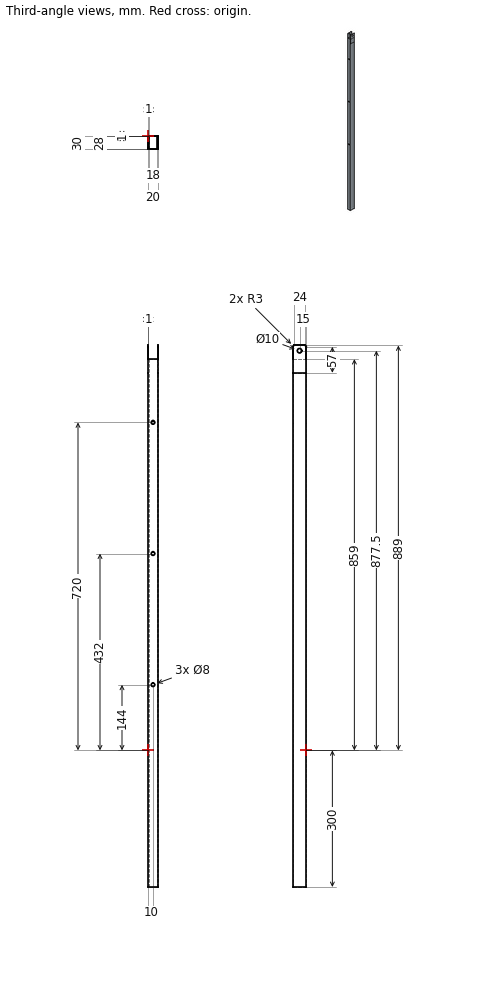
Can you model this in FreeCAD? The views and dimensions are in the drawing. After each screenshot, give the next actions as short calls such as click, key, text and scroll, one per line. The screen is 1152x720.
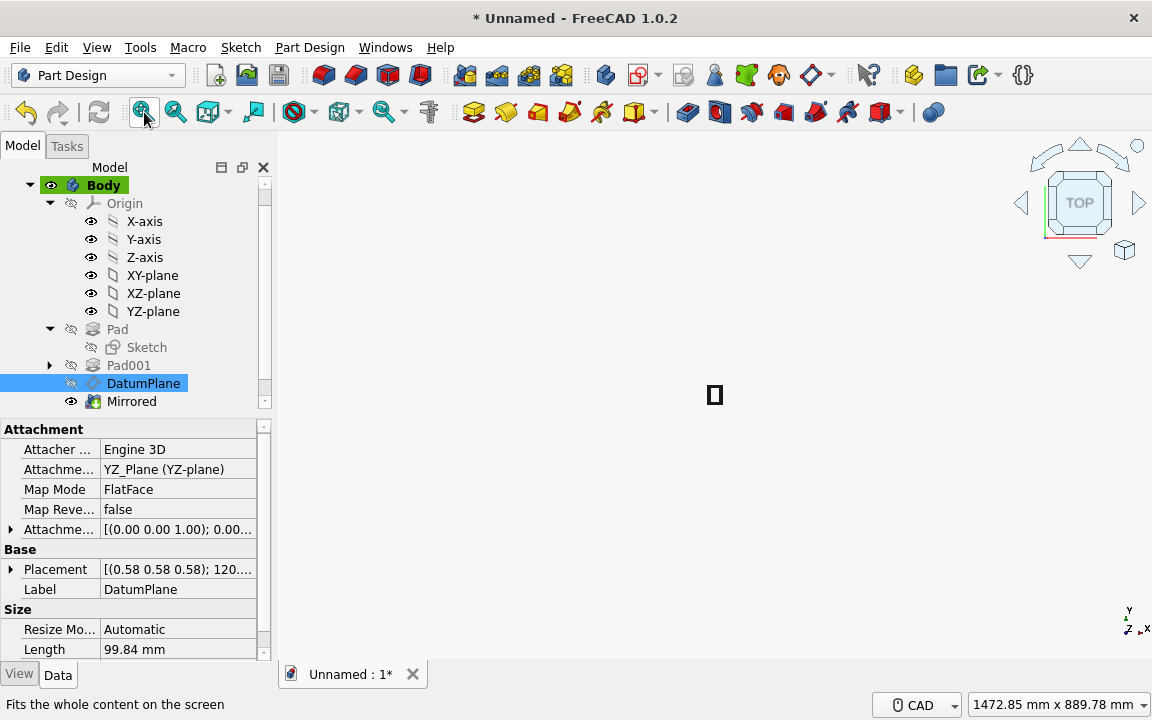
key(v)
key(f)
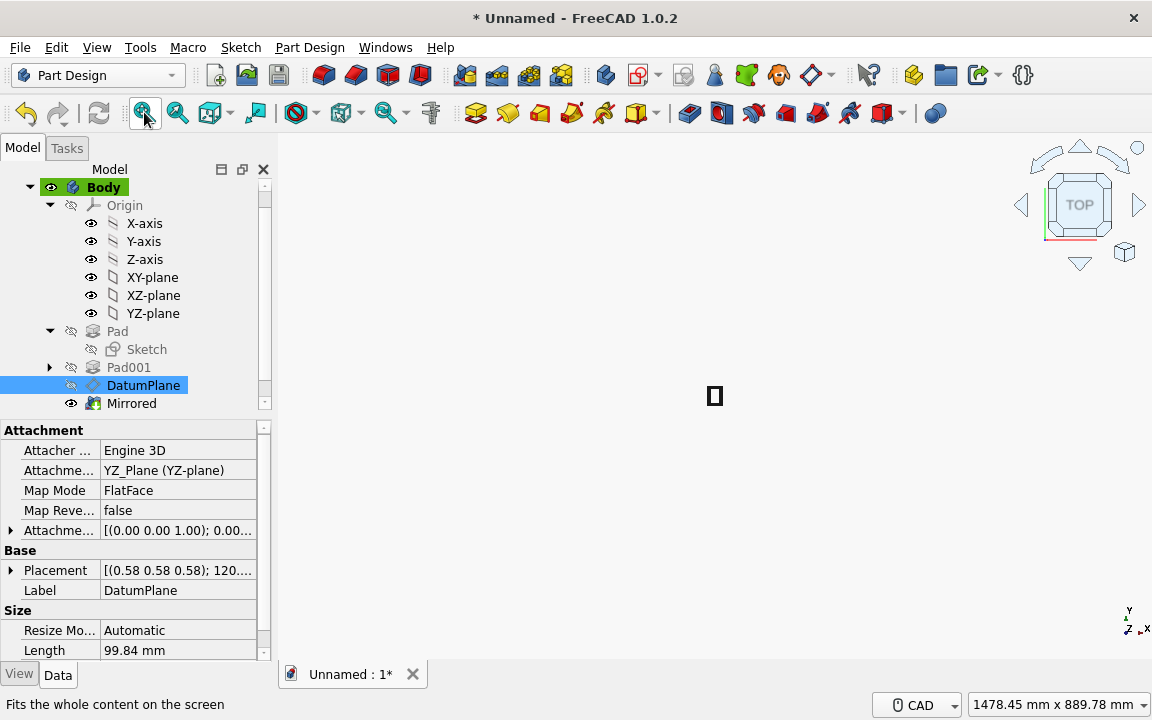
click(136, 313)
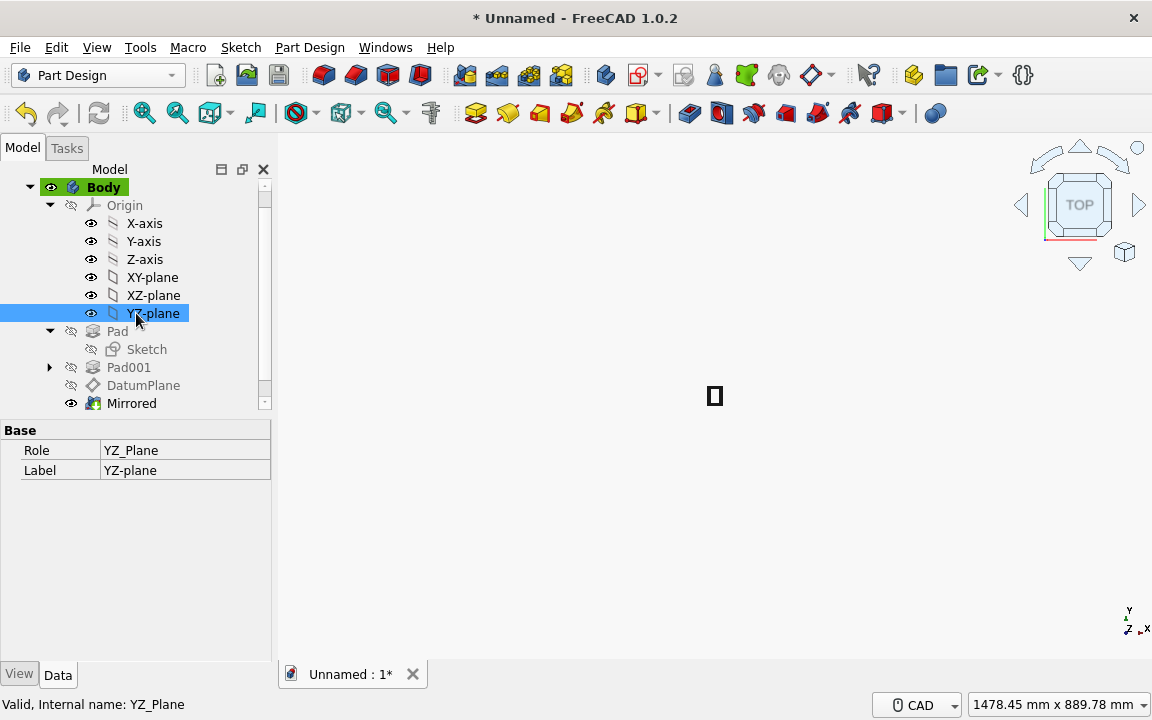
click(812, 76)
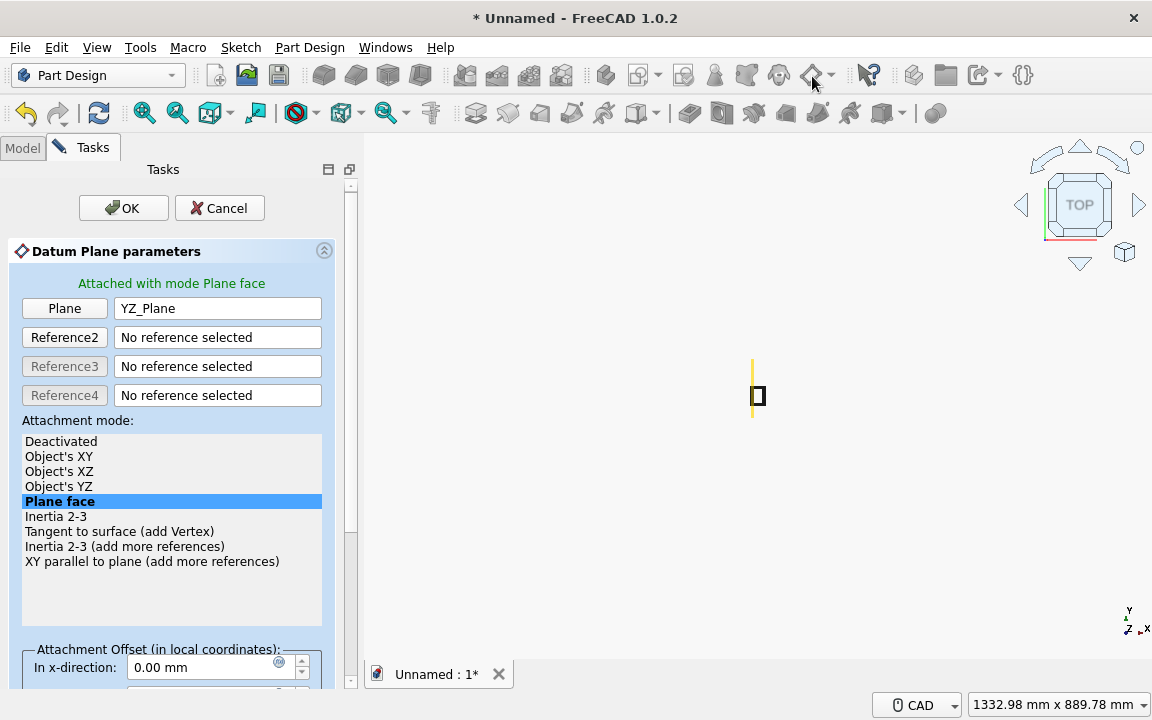
scroll(351, 434, down, 2)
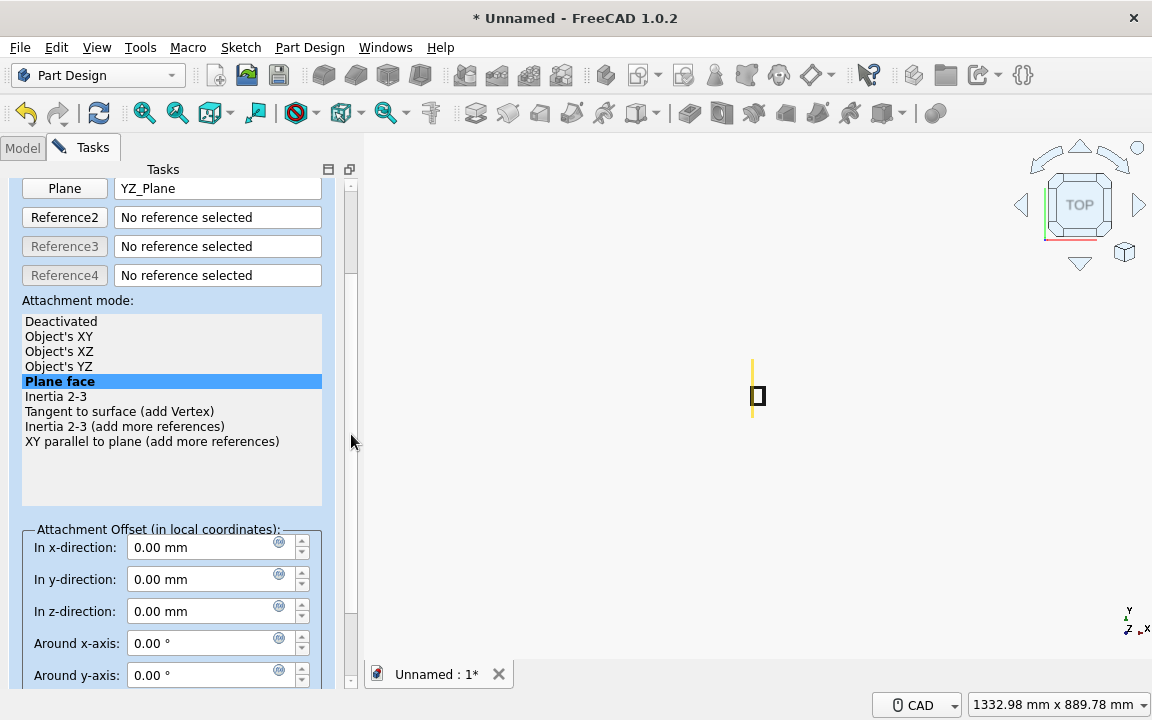
triple_click(210, 611)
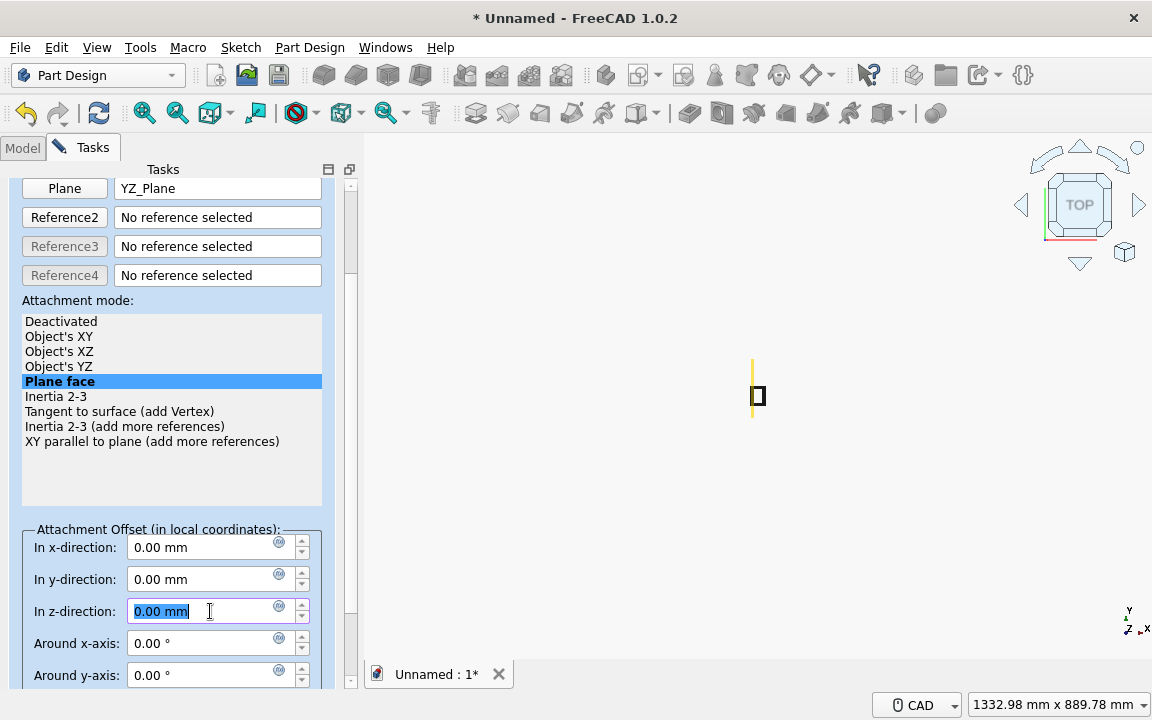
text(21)
key(Tab)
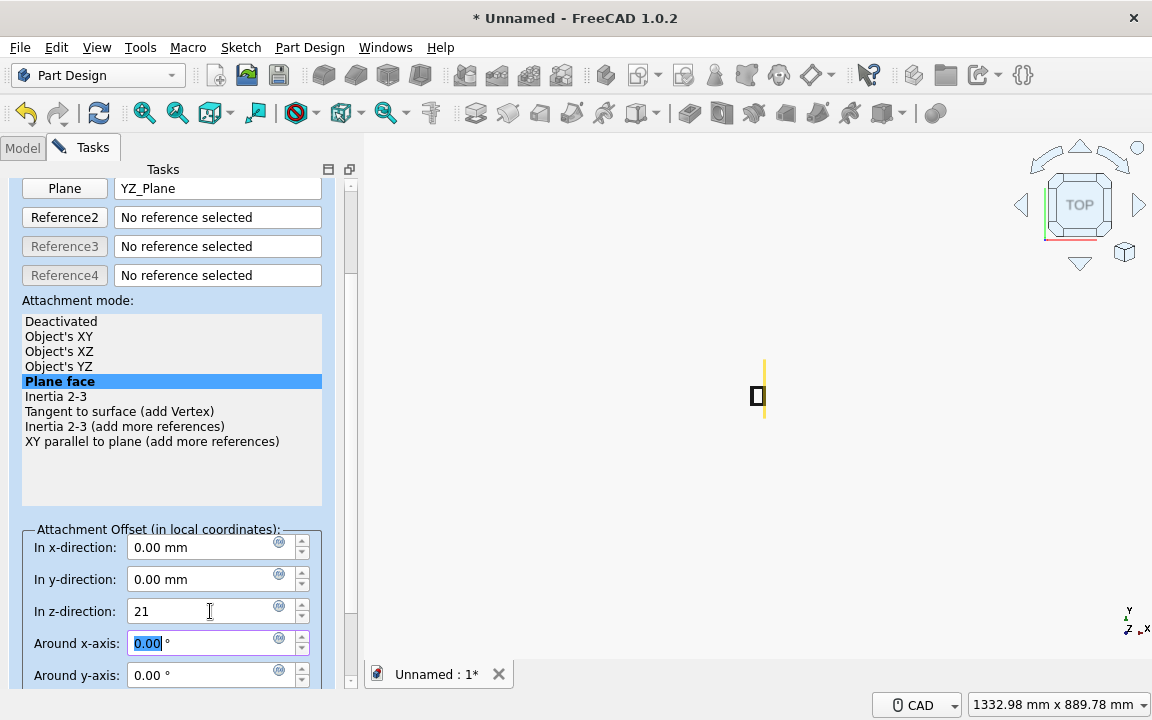
scroll(351, 434, up, 3)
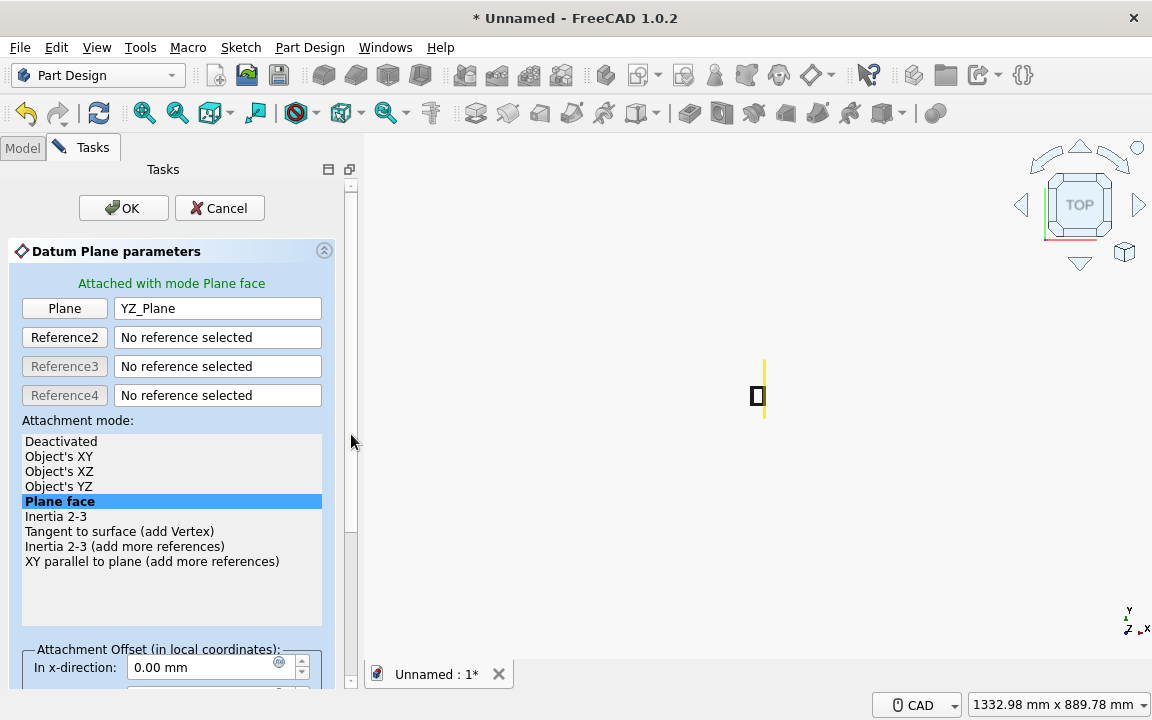
click(124, 208)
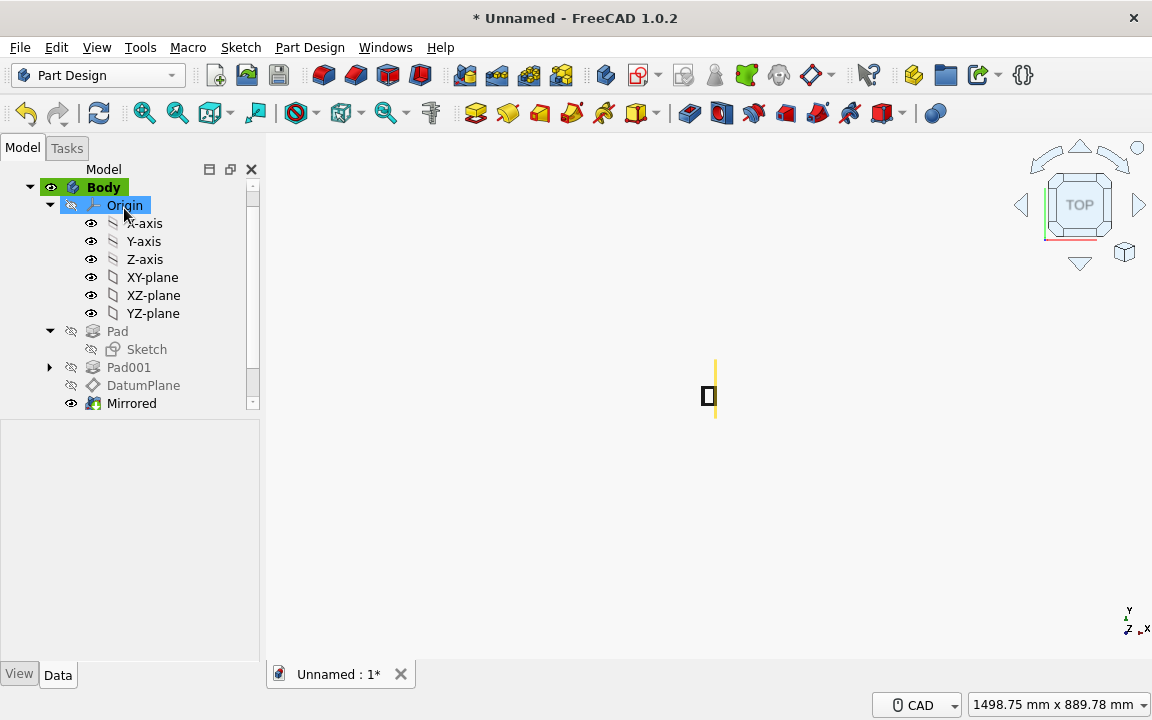
scroll(120, 291, down, 3)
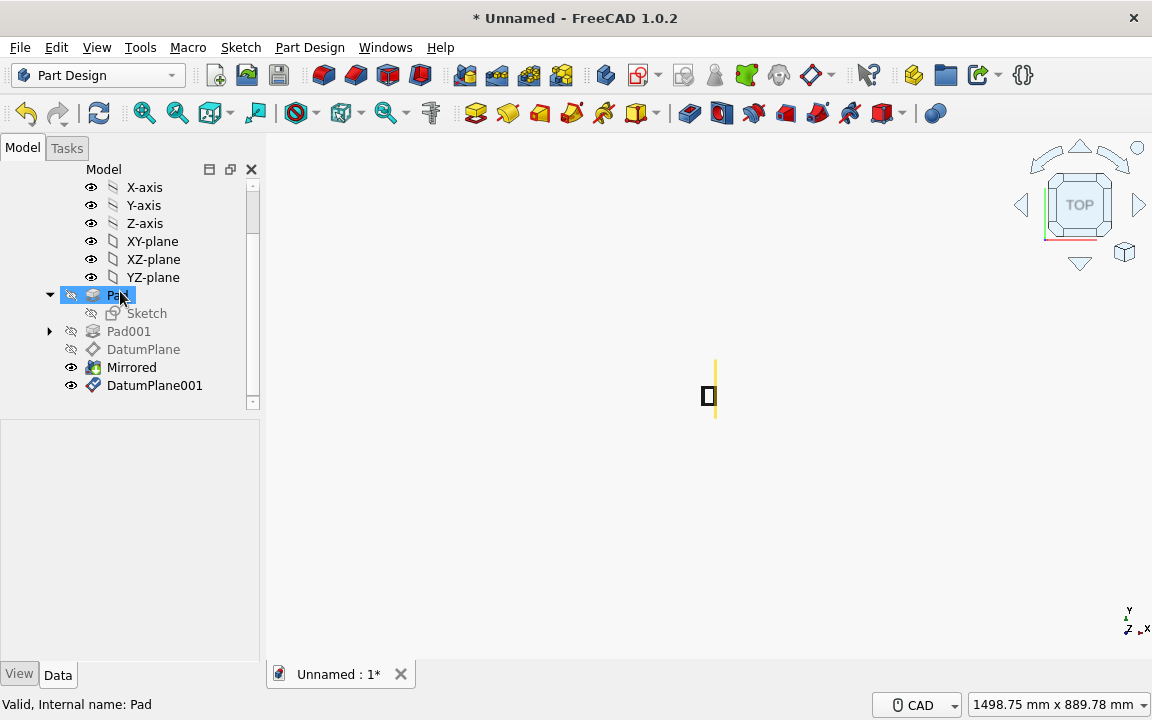
click(116, 385)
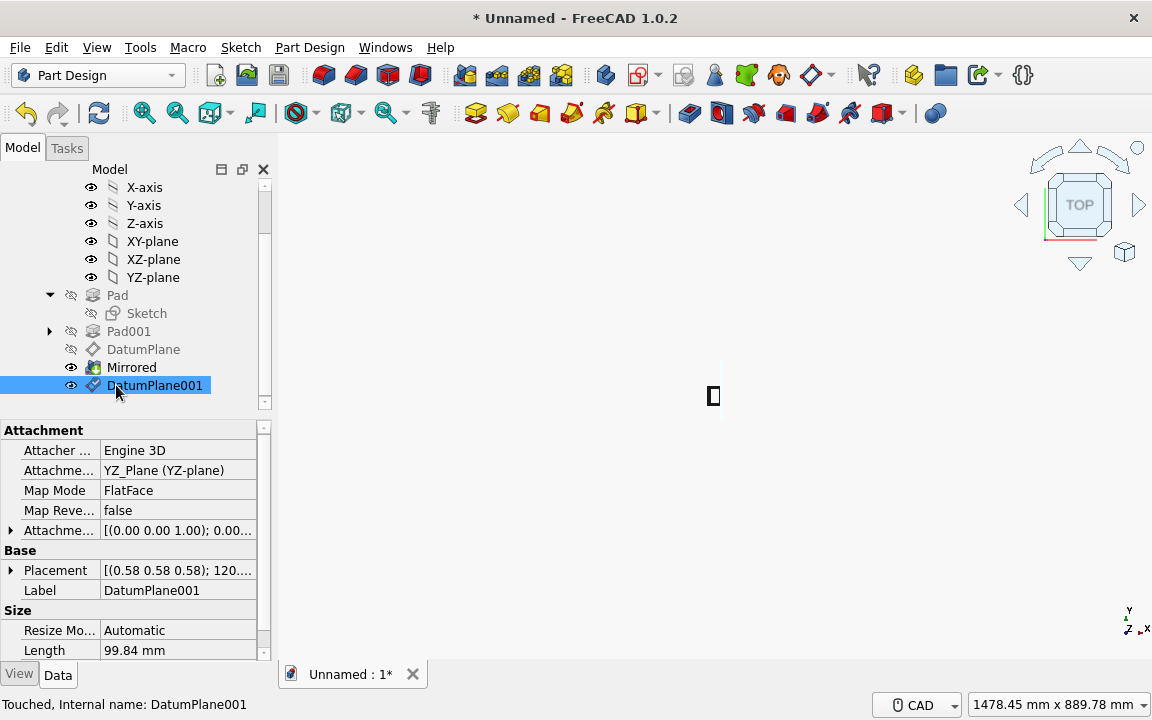
click(638, 76)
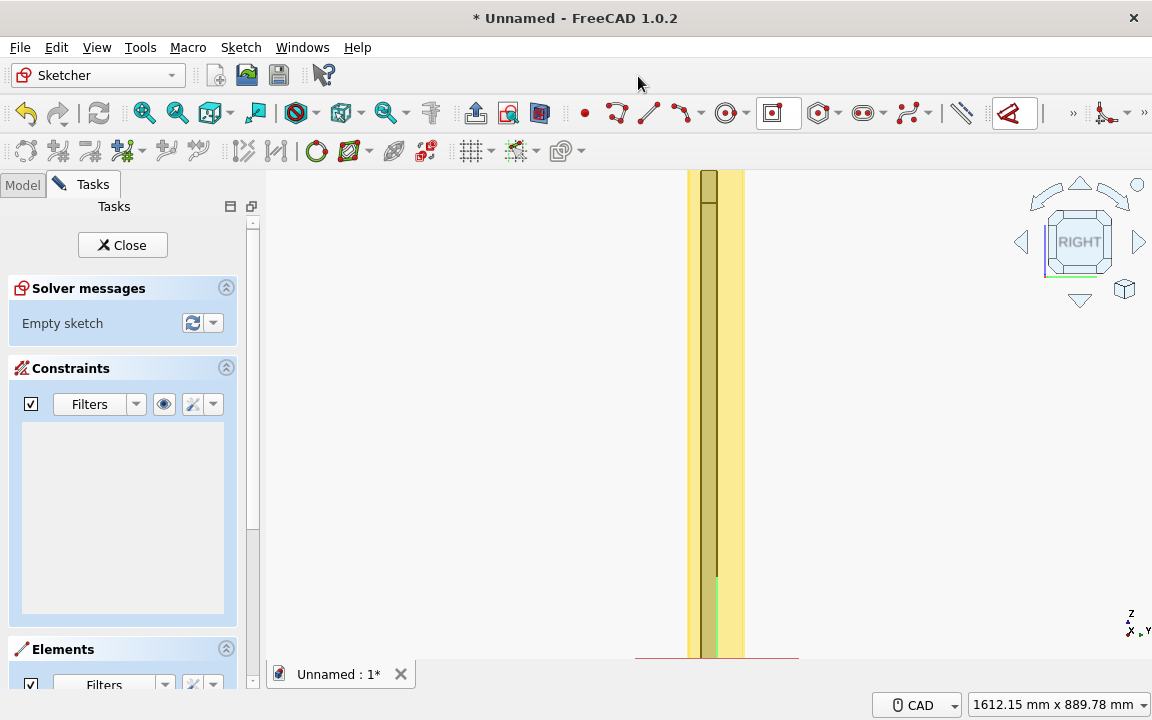
scroll(640, 414, down, 5)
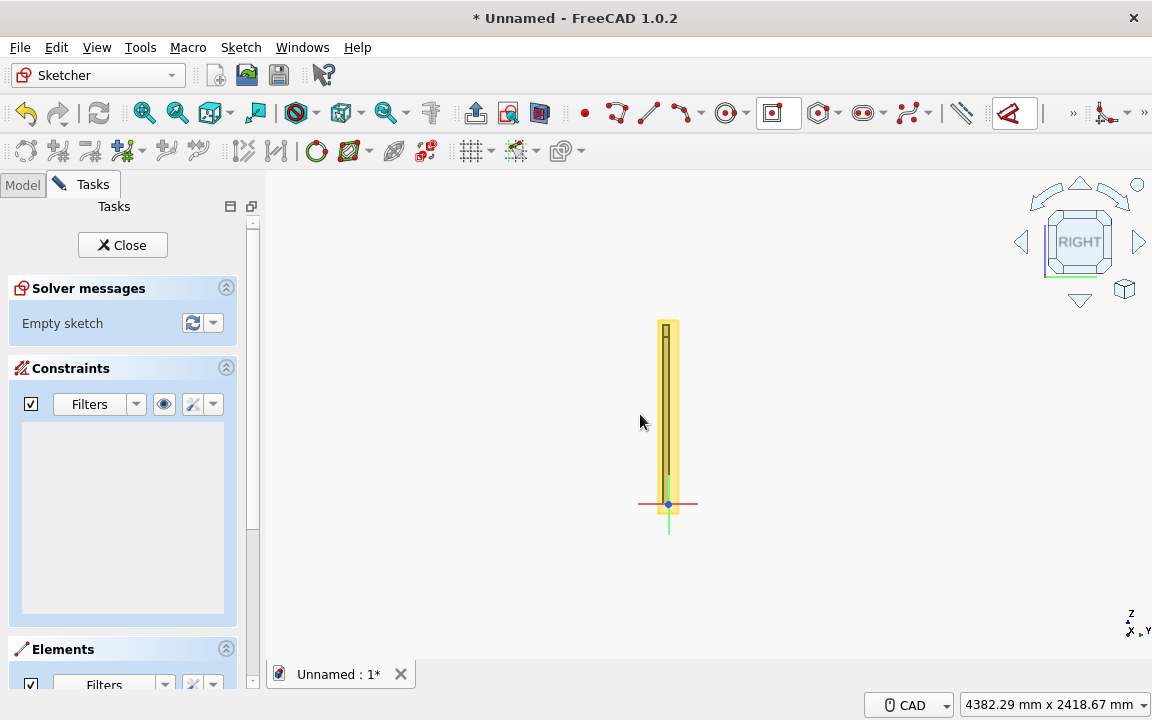
scroll(667, 322, up, 15)